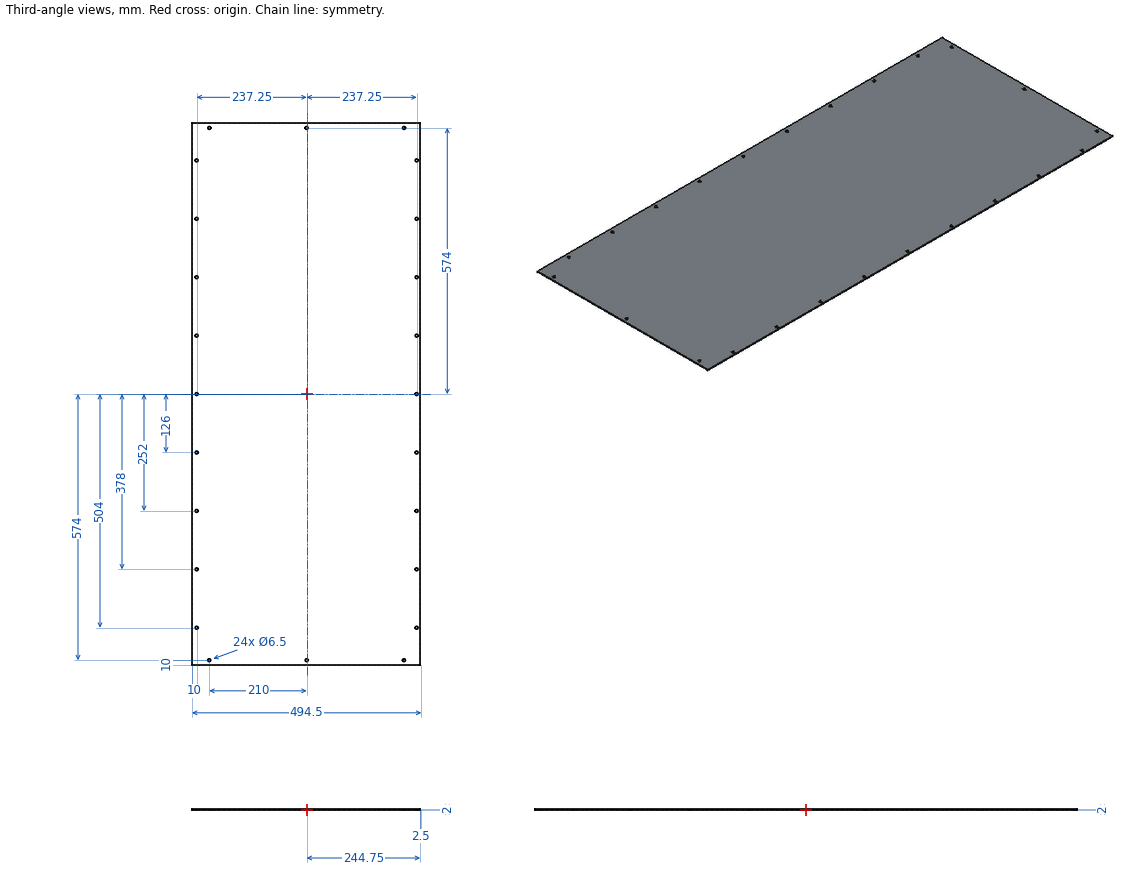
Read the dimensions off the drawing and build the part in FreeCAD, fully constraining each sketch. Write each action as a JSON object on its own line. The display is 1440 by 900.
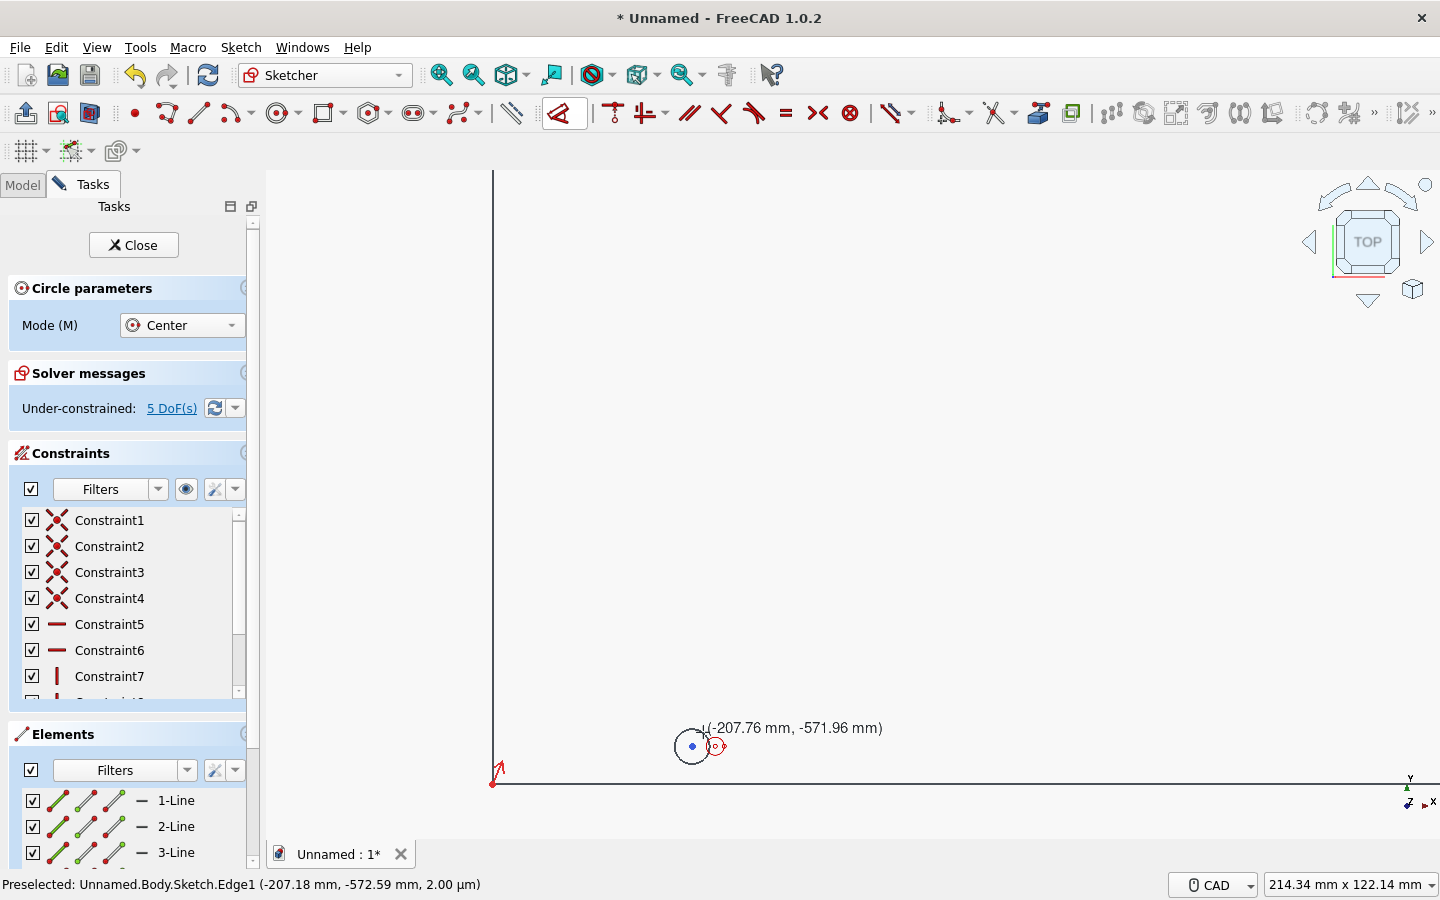
{"action": "scroll", "coordinate": [541, 361], "scroll_direction": "up", "scroll_amount": 2}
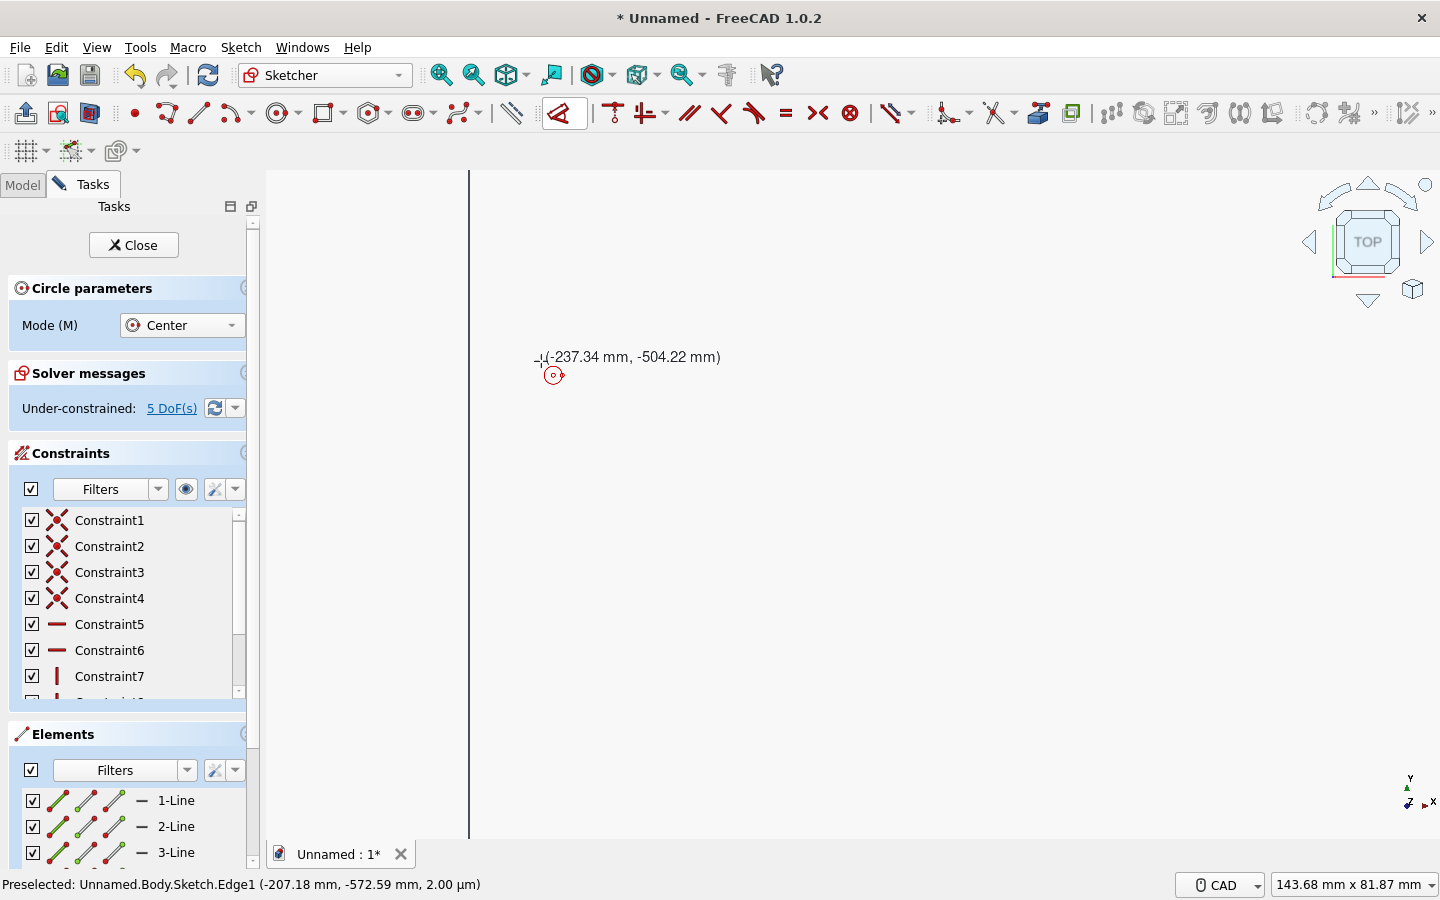
{"action": "scroll", "coordinate": [696, 728], "scroll_direction": "down", "scroll_amount": 15}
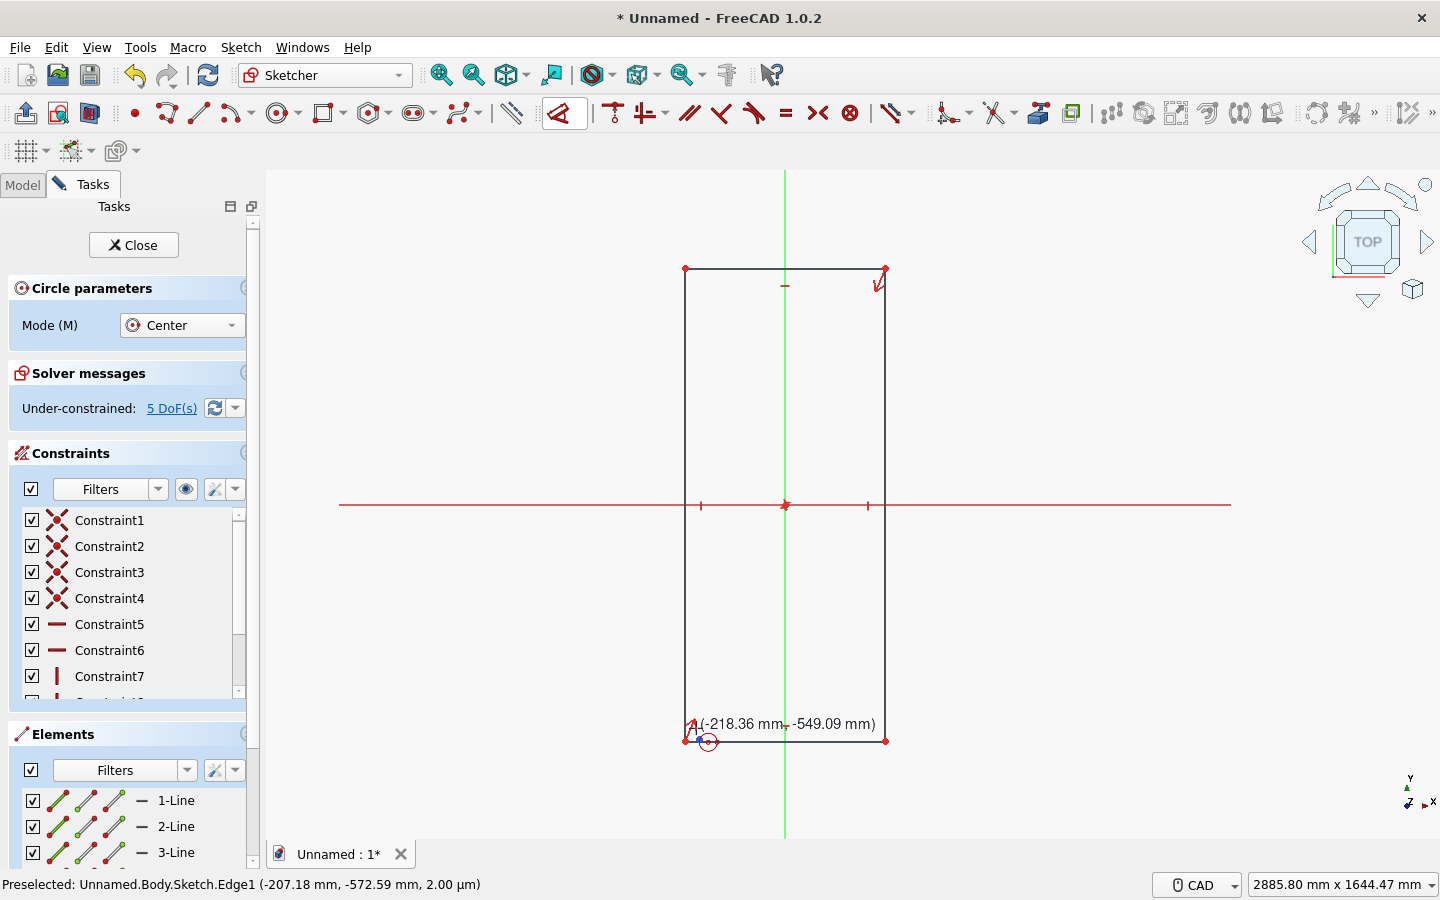
{"action": "scroll", "coordinate": [689, 710], "scroll_direction": "up", "scroll_amount": 7}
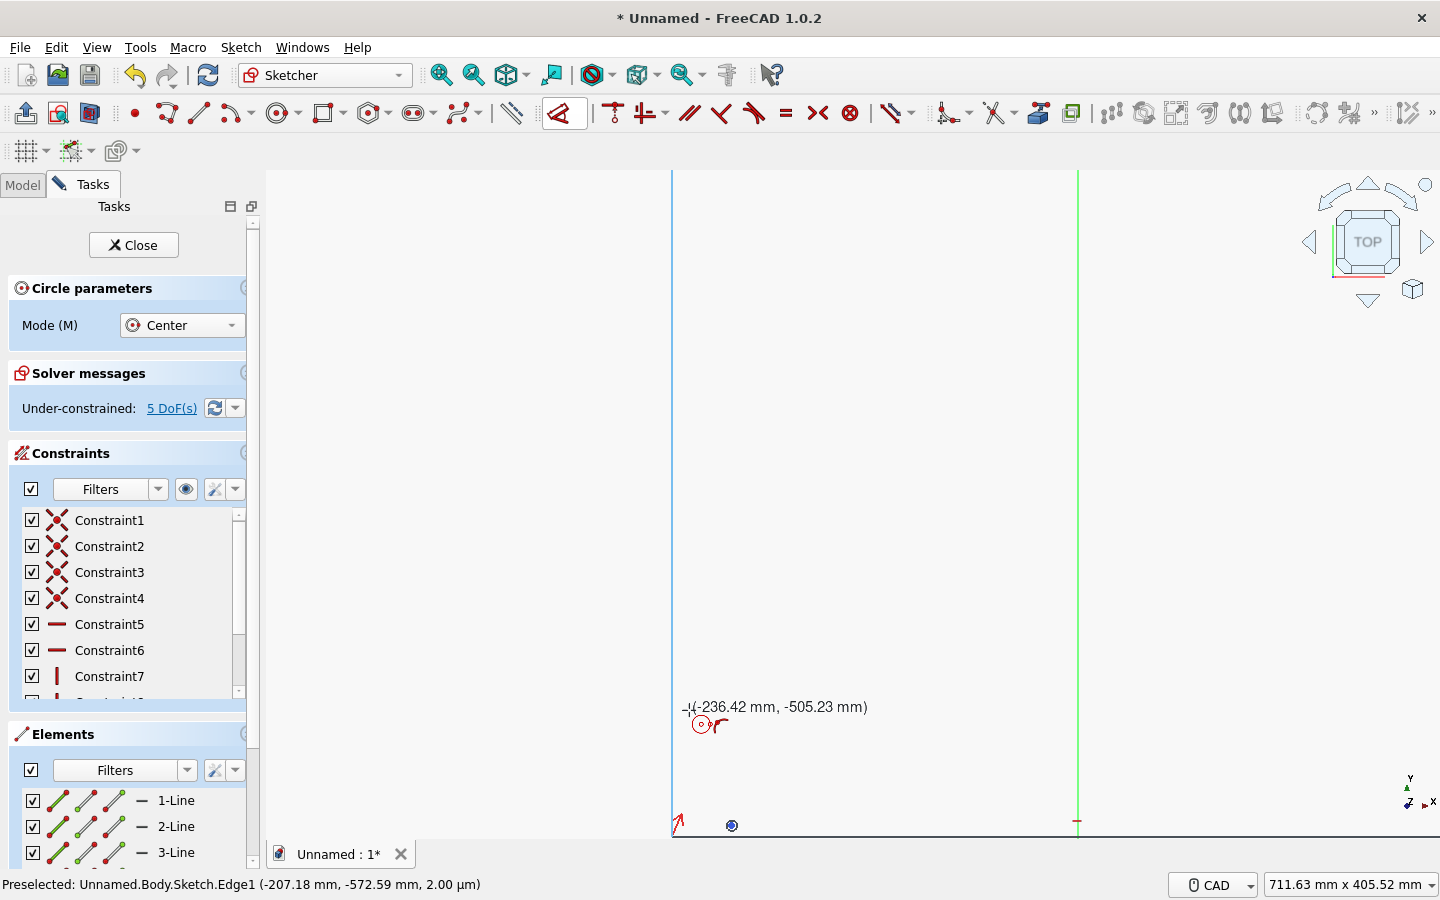
{"action": "left_click", "coordinate": [687, 710]}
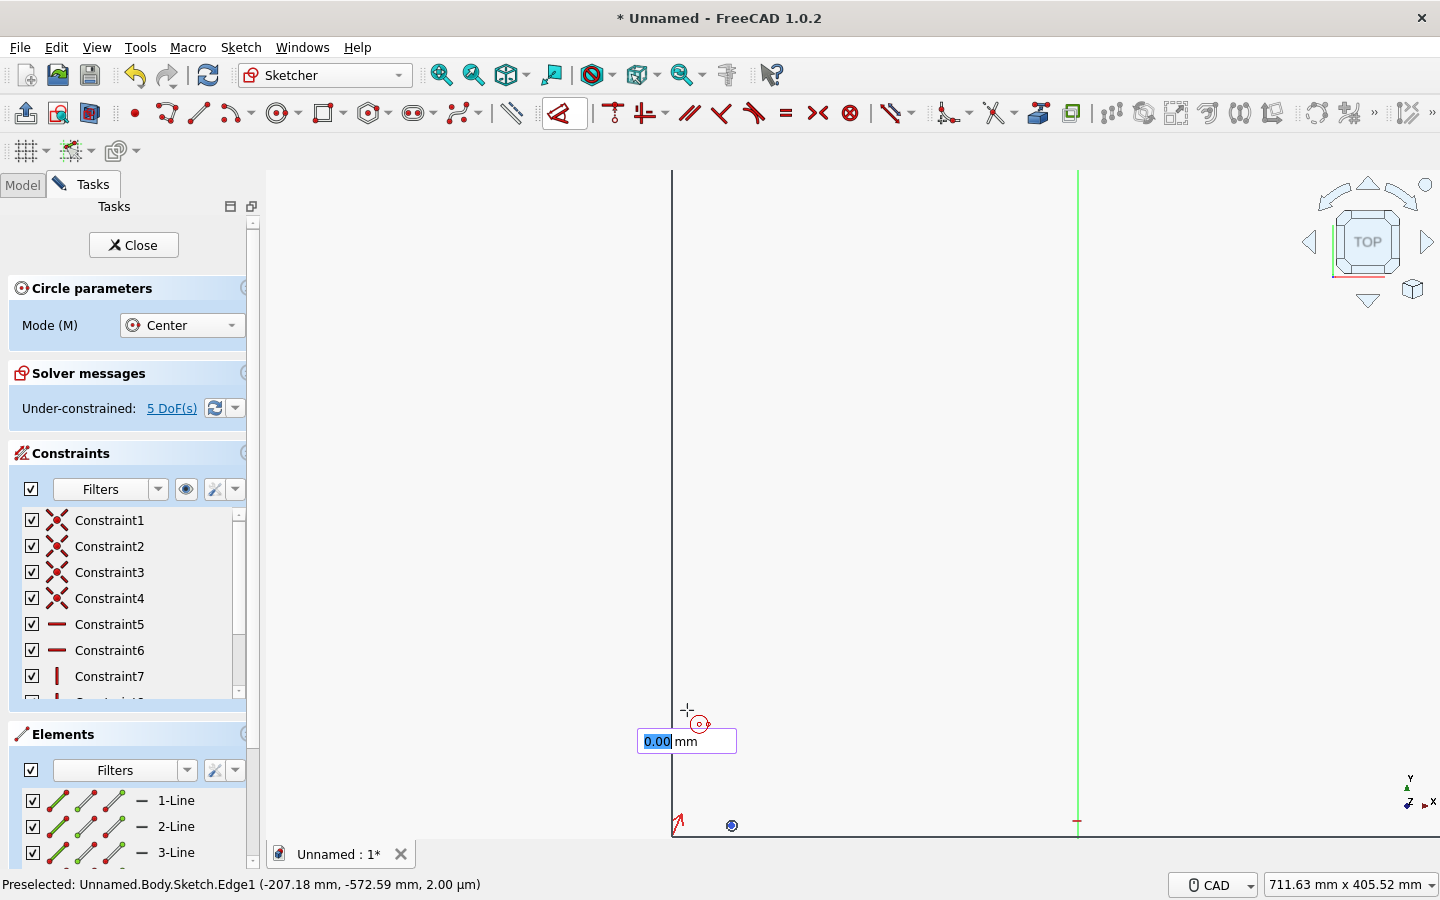
{"action": "scroll", "coordinate": [690, 706], "scroll_direction": "up", "scroll_amount": 6}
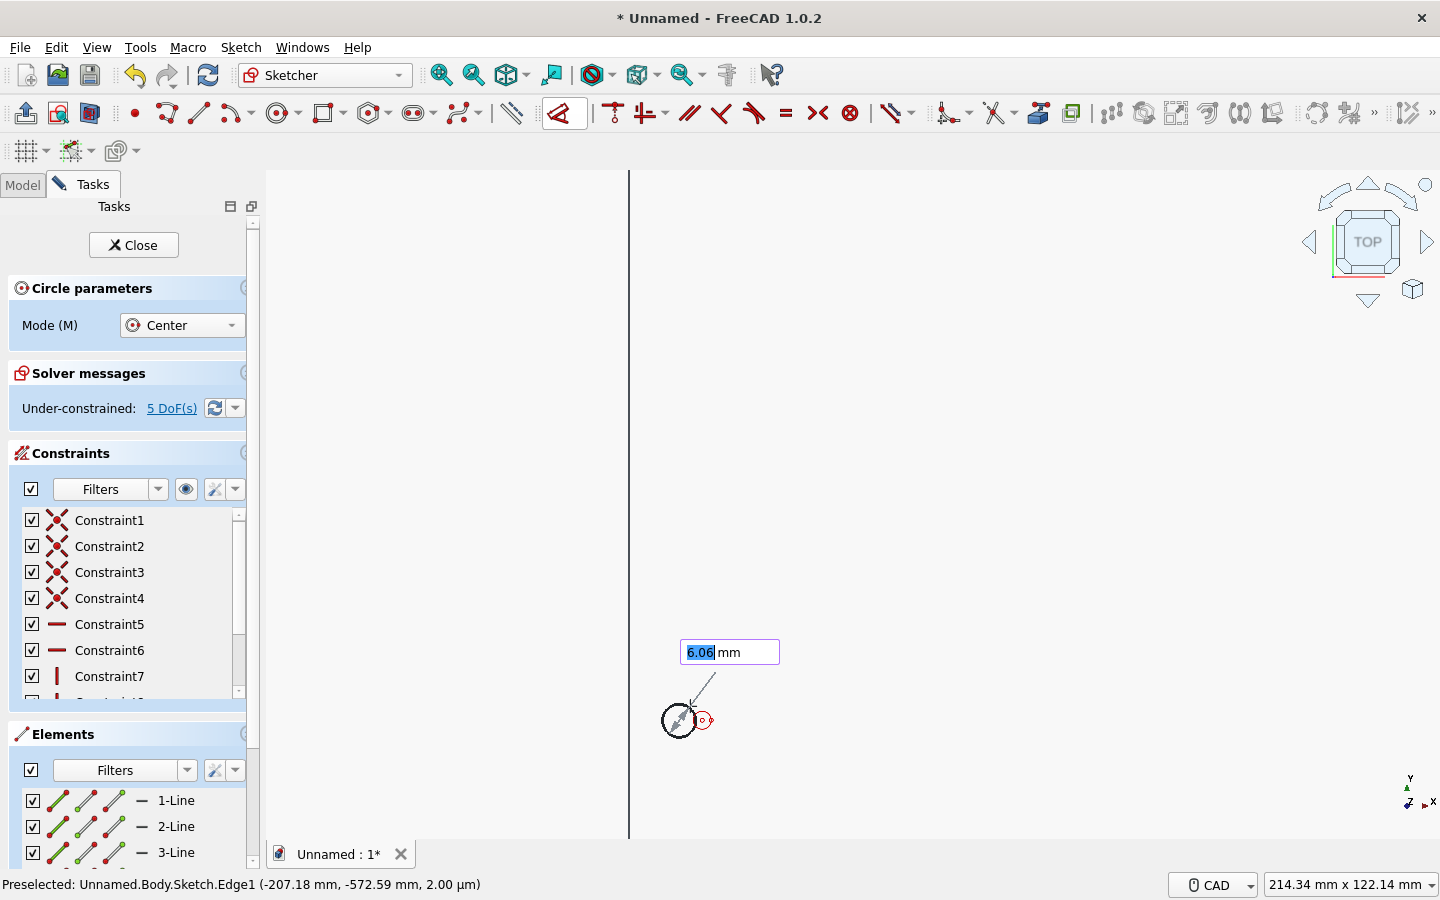
{"action": "left_click", "coordinate": [690, 703]}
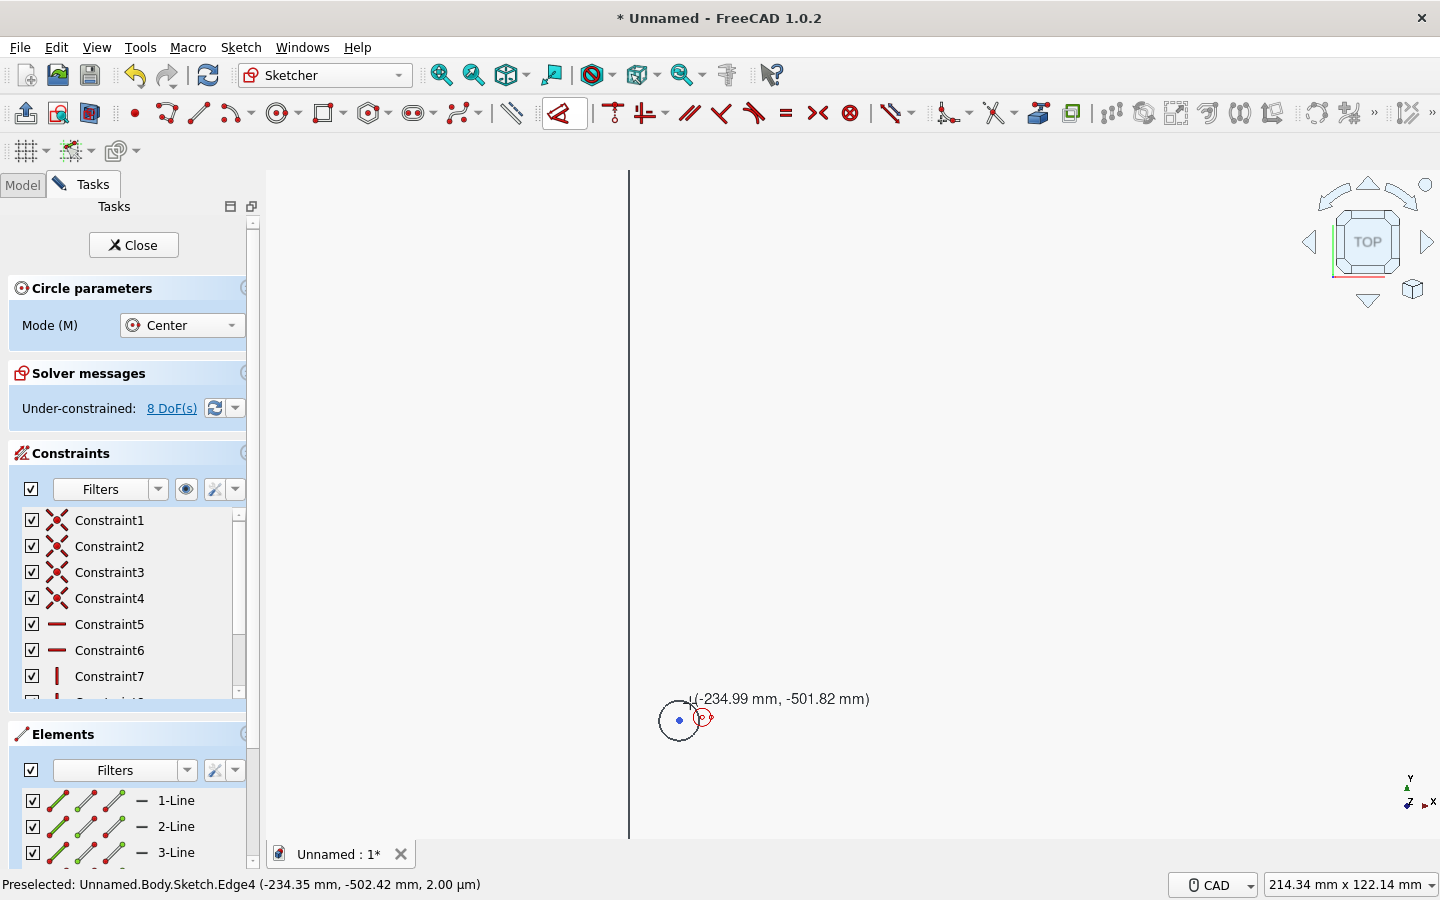
{"action": "scroll", "coordinate": [689, 709], "scroll_direction": "down", "scroll_amount": 13}